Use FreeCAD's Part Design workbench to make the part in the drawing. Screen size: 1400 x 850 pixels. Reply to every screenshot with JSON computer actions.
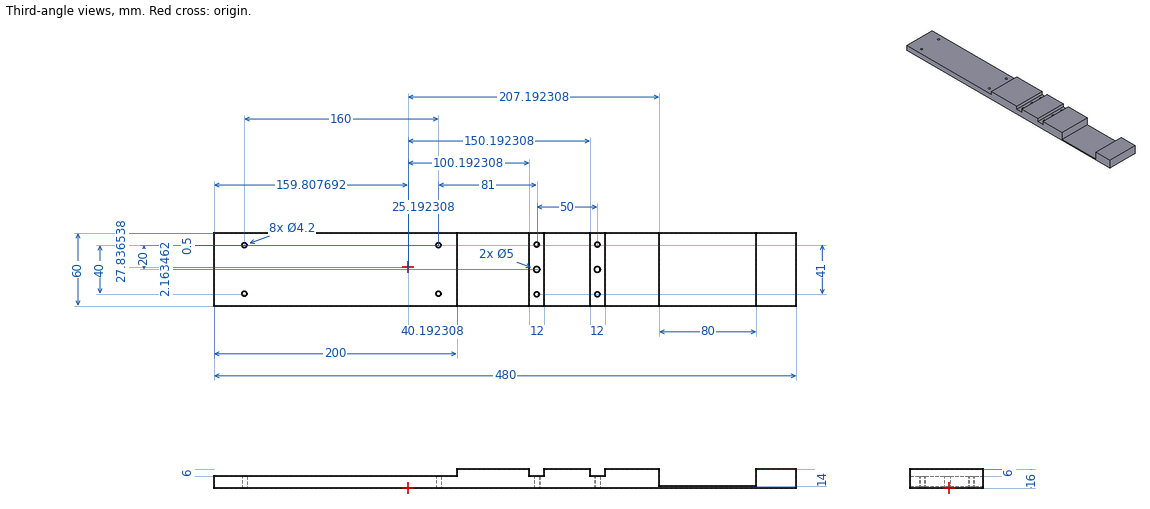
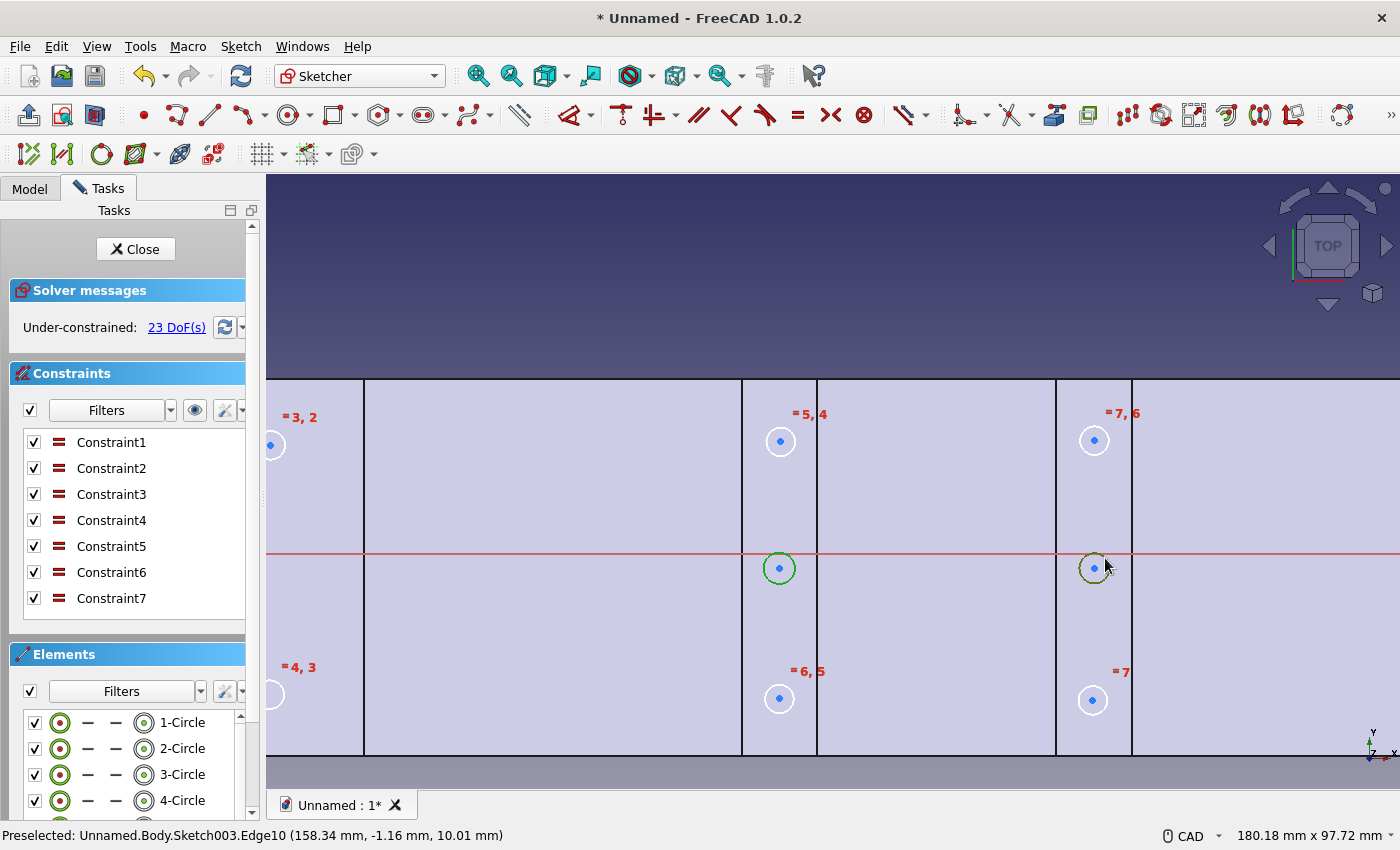
{"action": "key", "text": "e"}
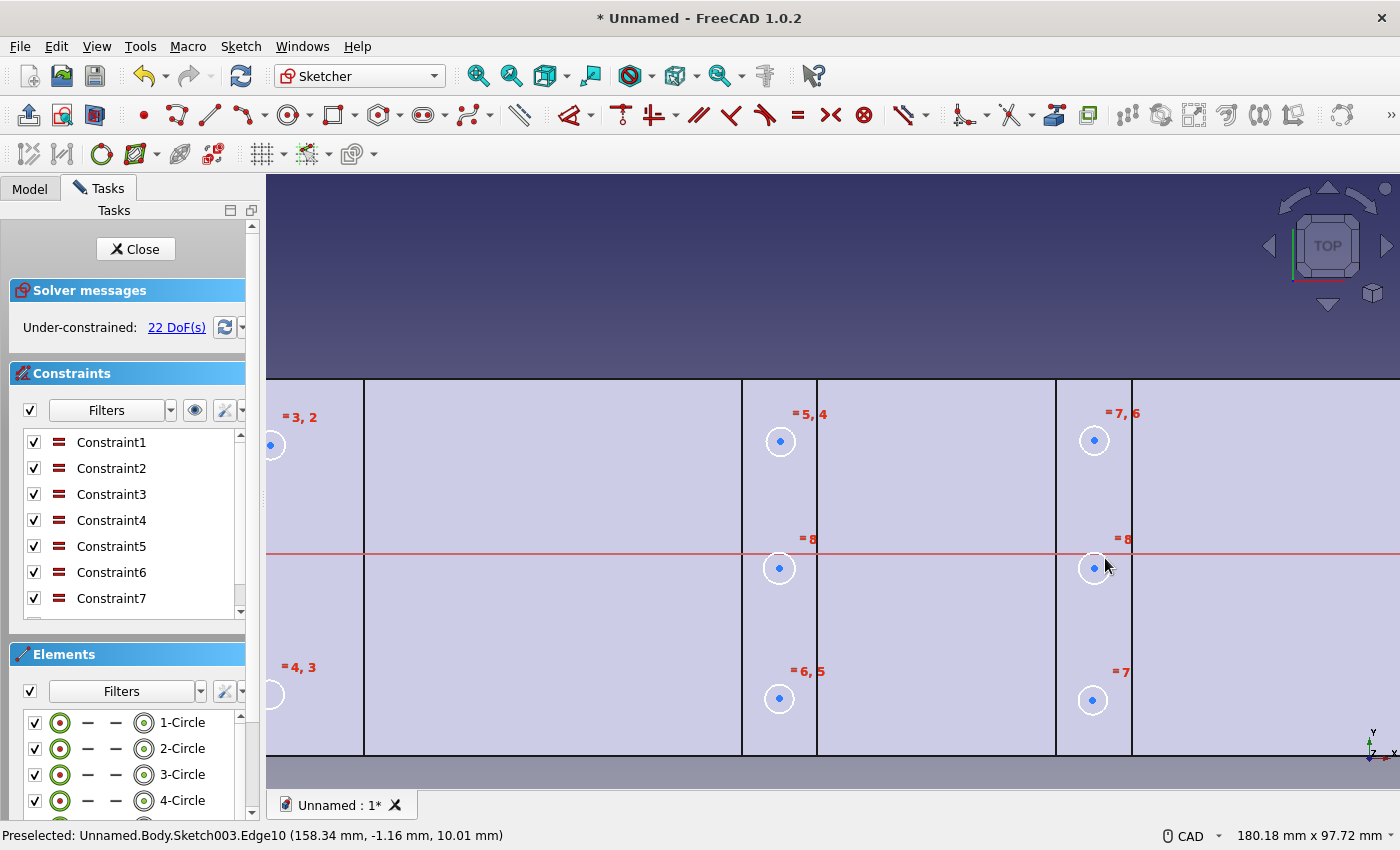
{"action": "scroll", "coordinate": [1105, 432], "scroll_direction": "down", "scroll_amount": 5}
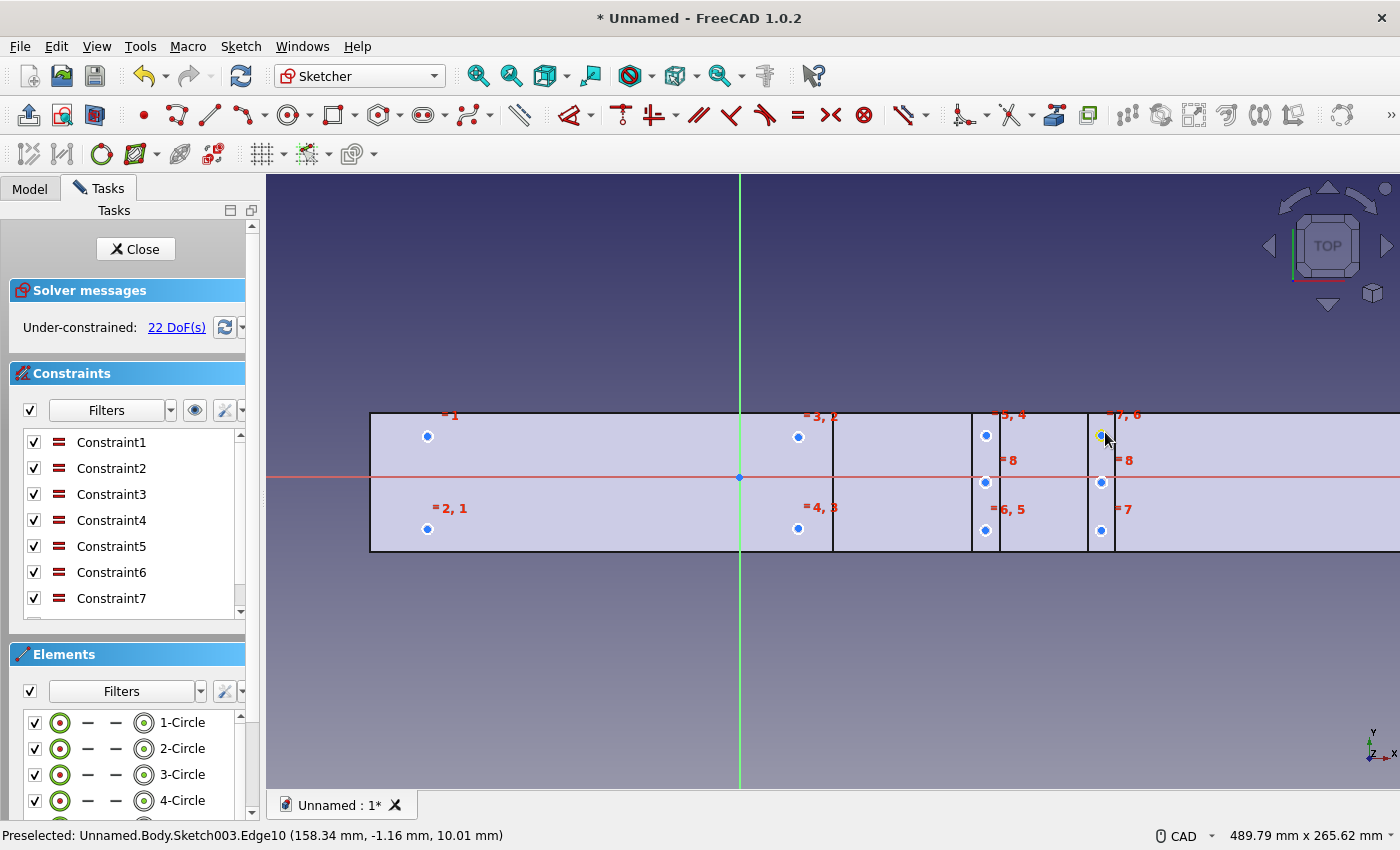
{"action": "left_click", "coordinate": [428, 437]}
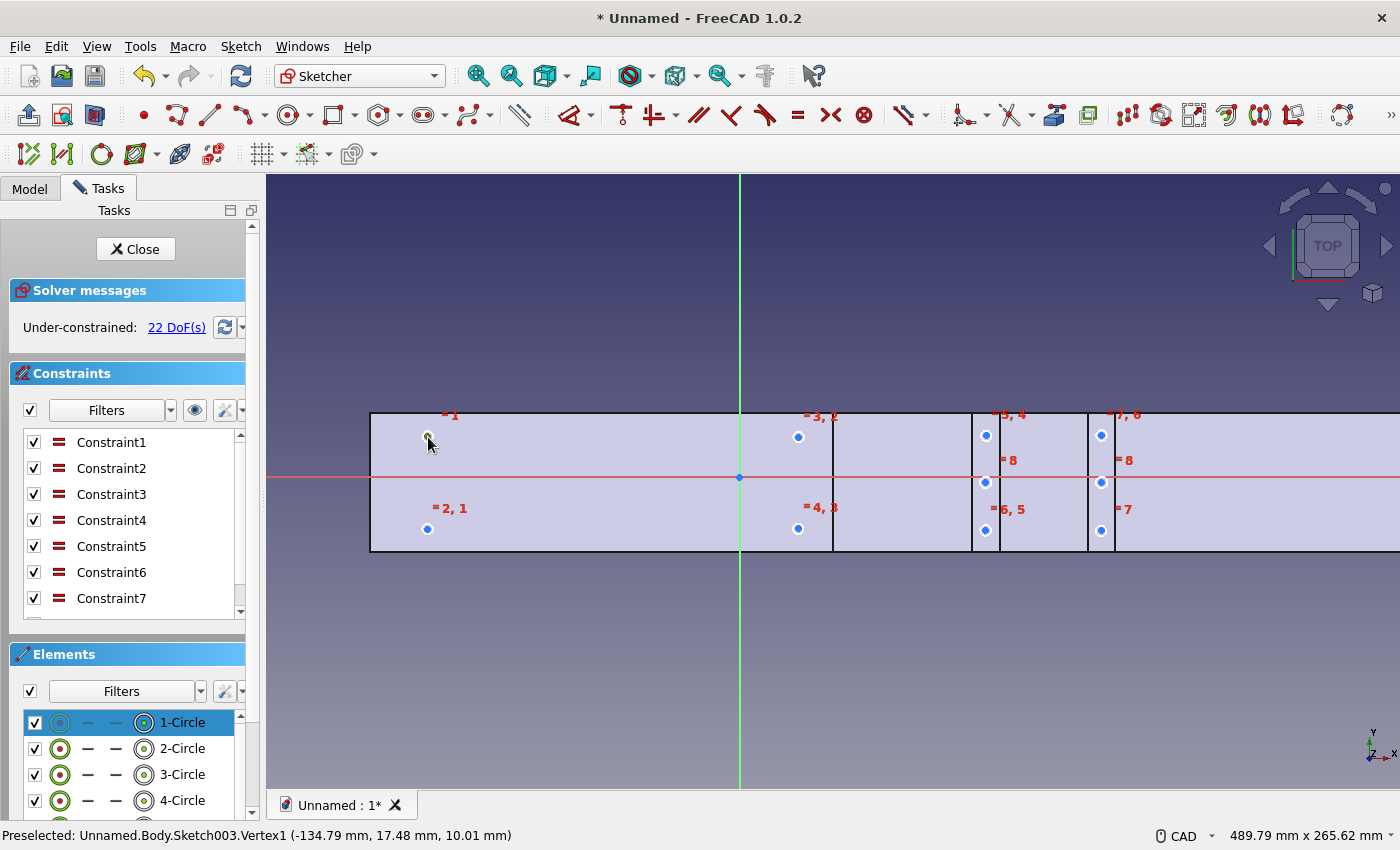
{"action": "left_click", "coordinate": [428, 529]}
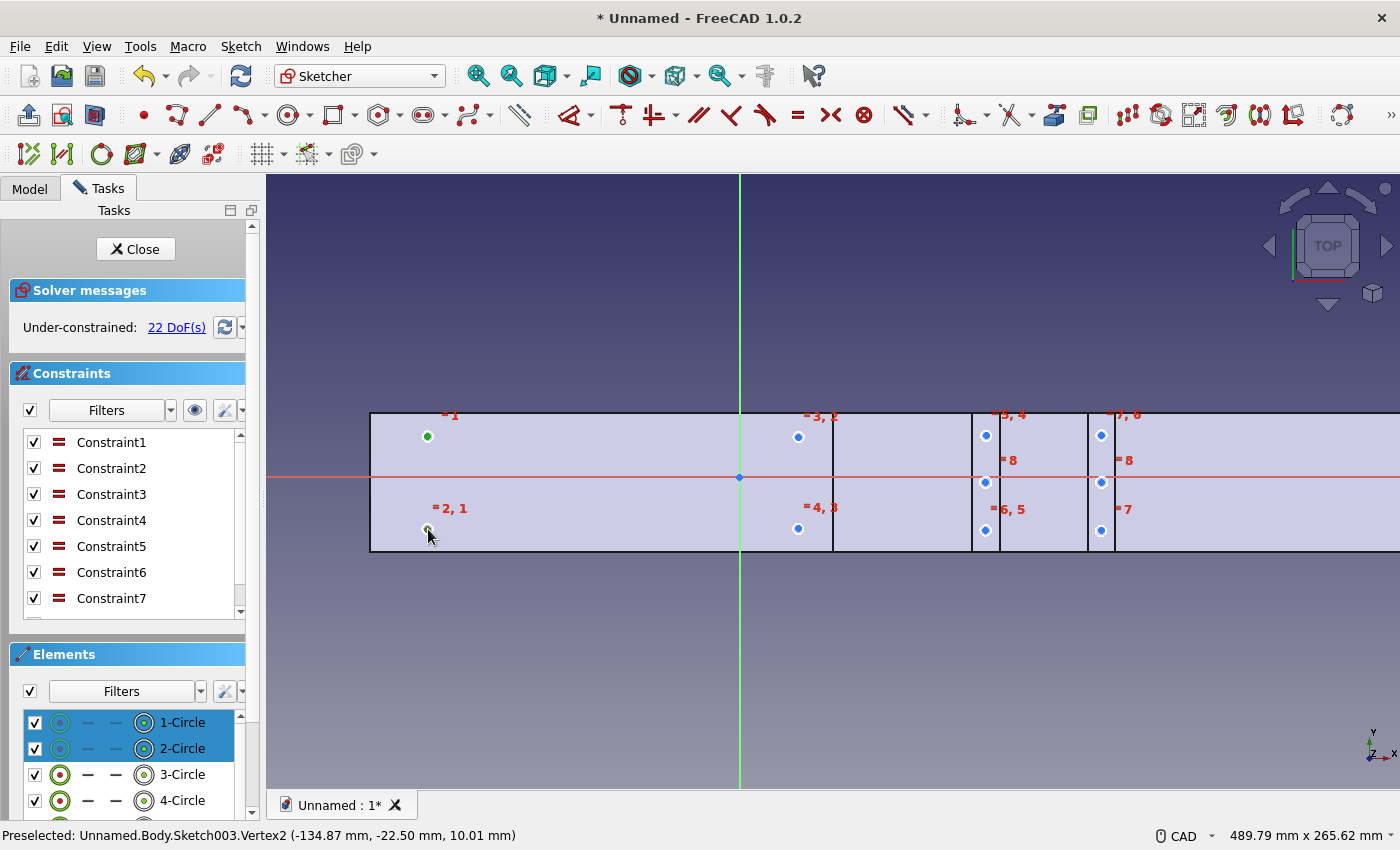
{"action": "key", "text": "v"}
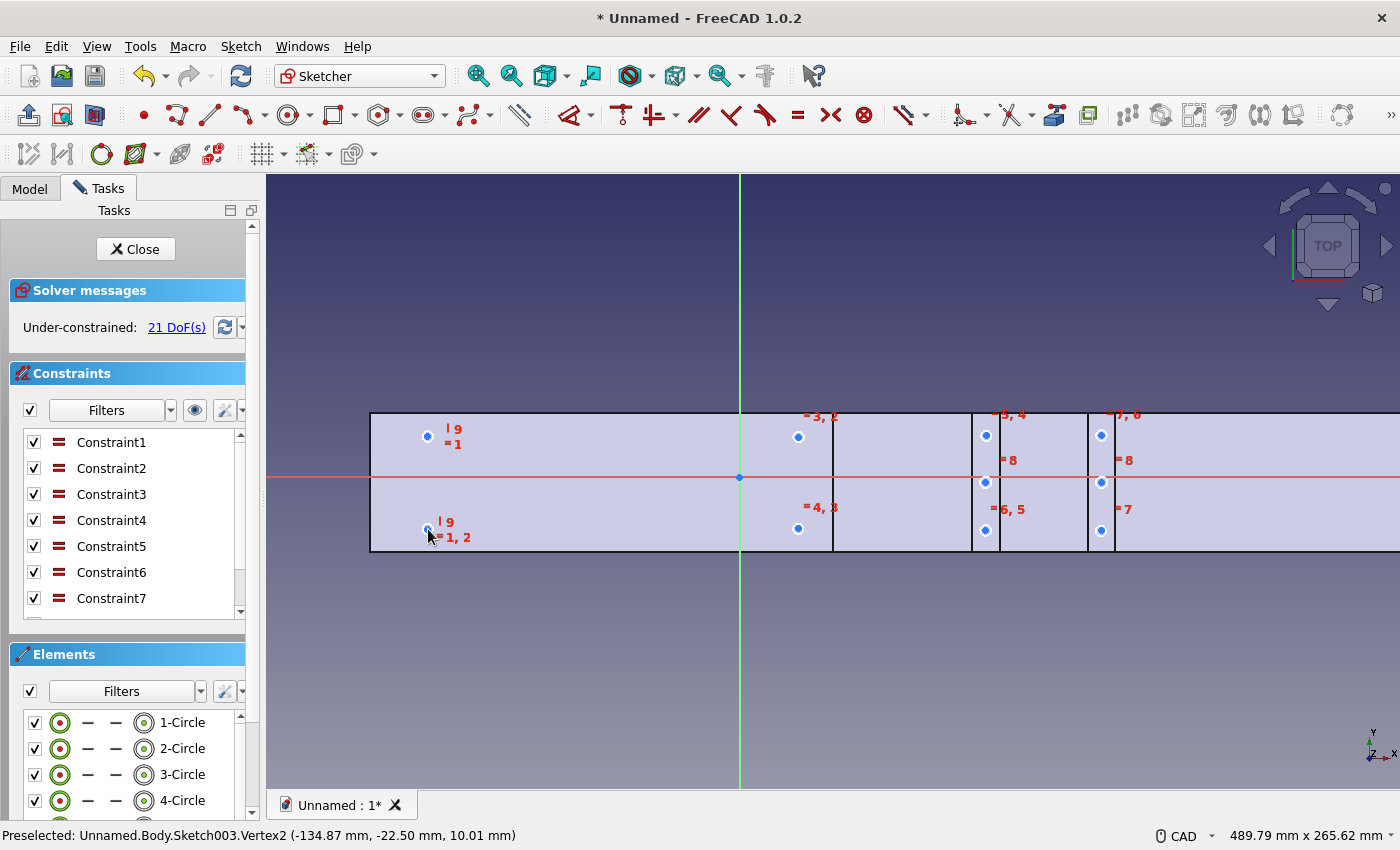
{"action": "left_click", "coordinate": [428, 437]}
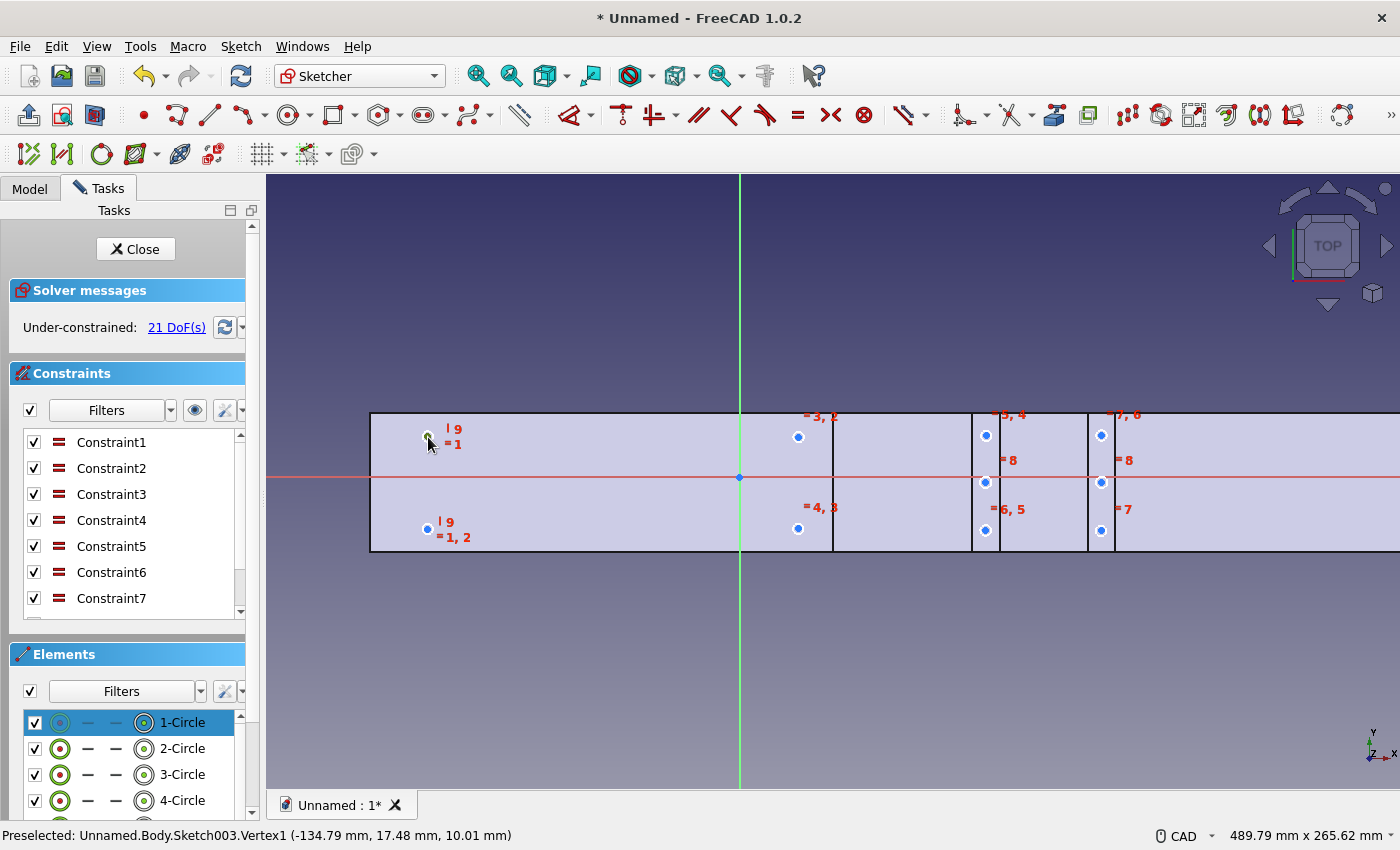
{"action": "left_click", "coordinate": [799, 437]}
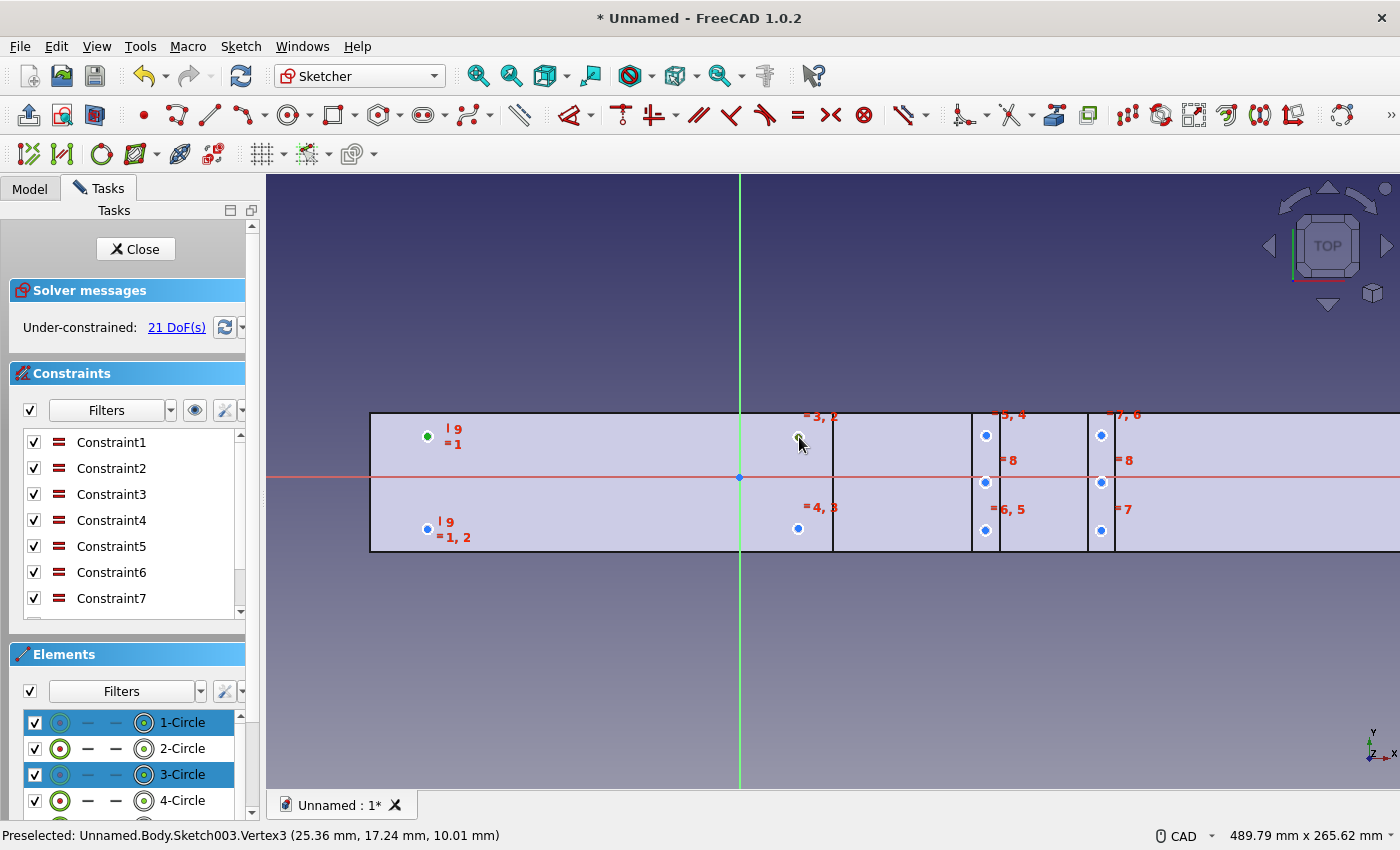
{"action": "left_click", "coordinate": [676, 116]}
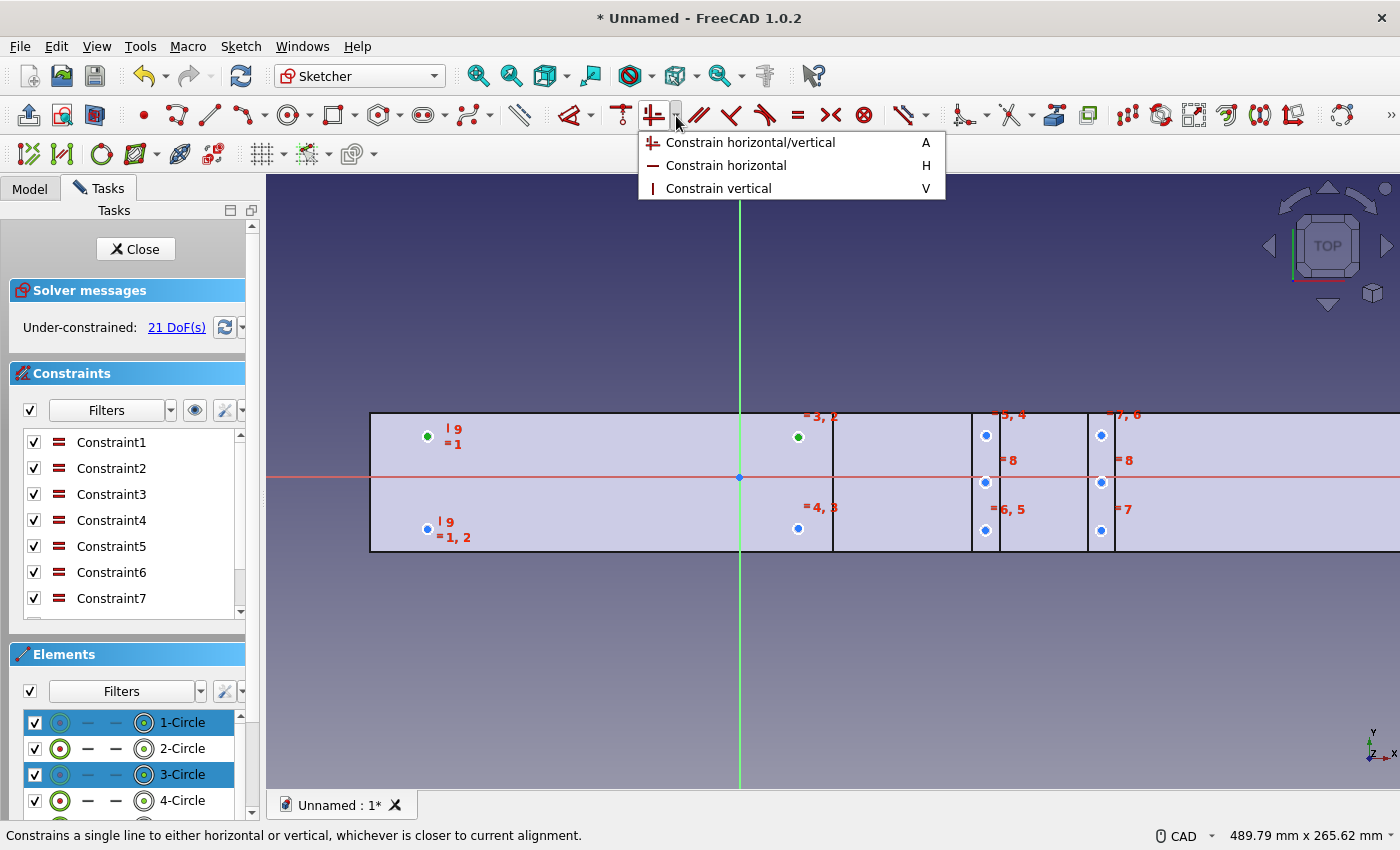
{"action": "left_click", "coordinate": [792, 166]}